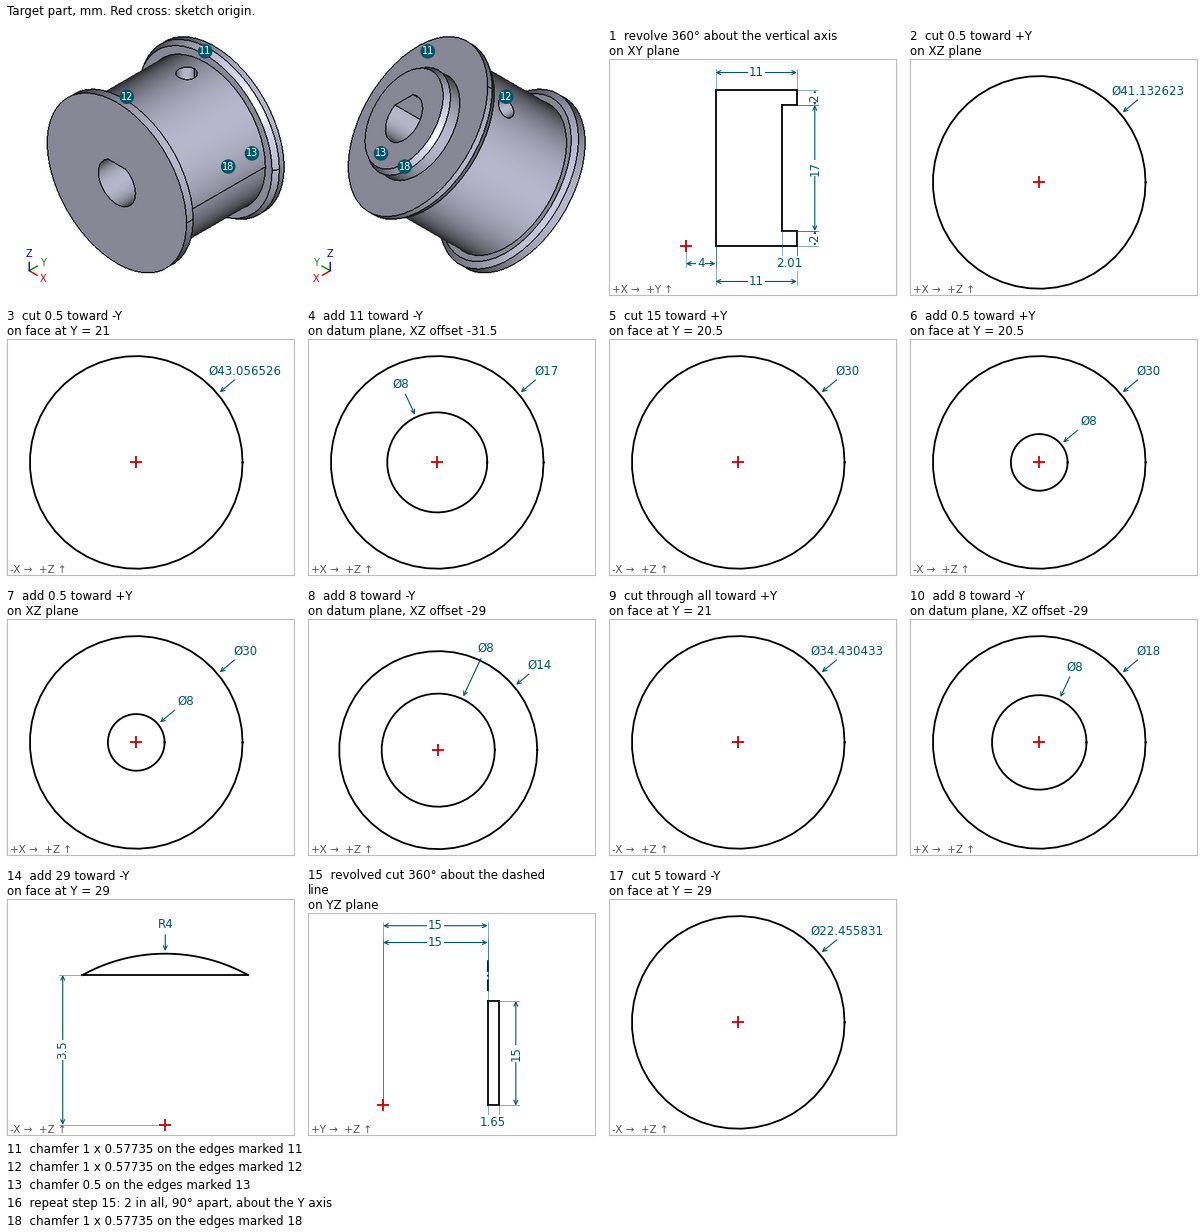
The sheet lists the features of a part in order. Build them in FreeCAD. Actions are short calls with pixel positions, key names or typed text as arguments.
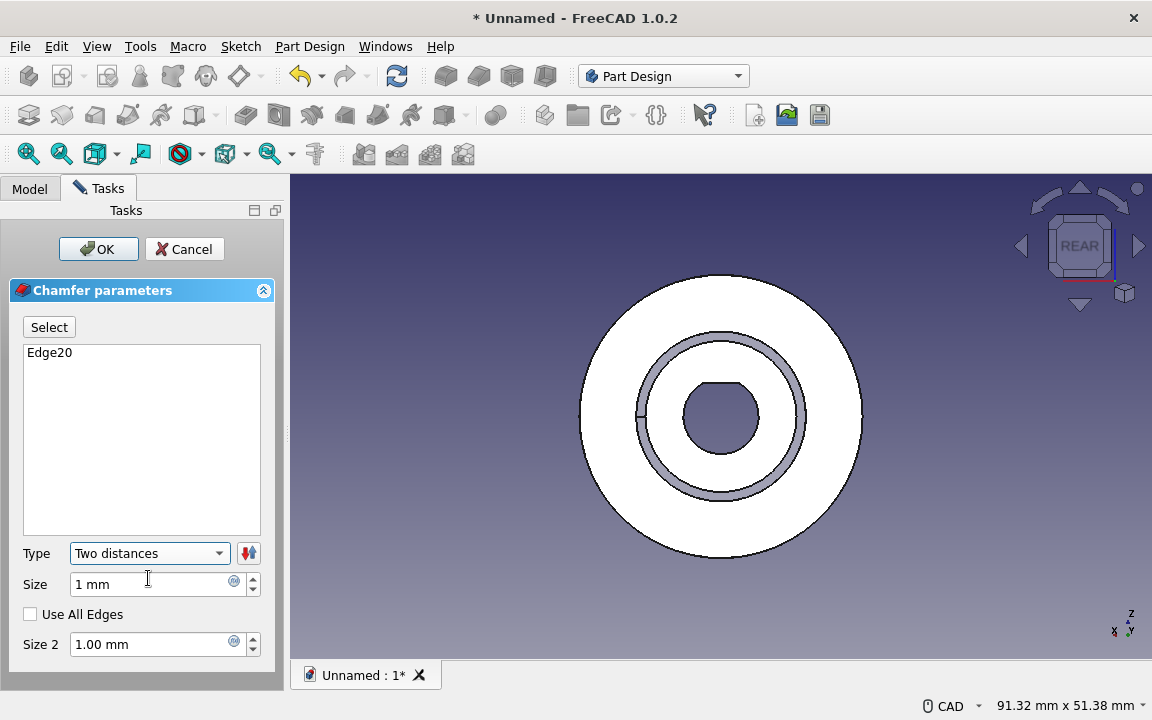
triple_click(158, 644)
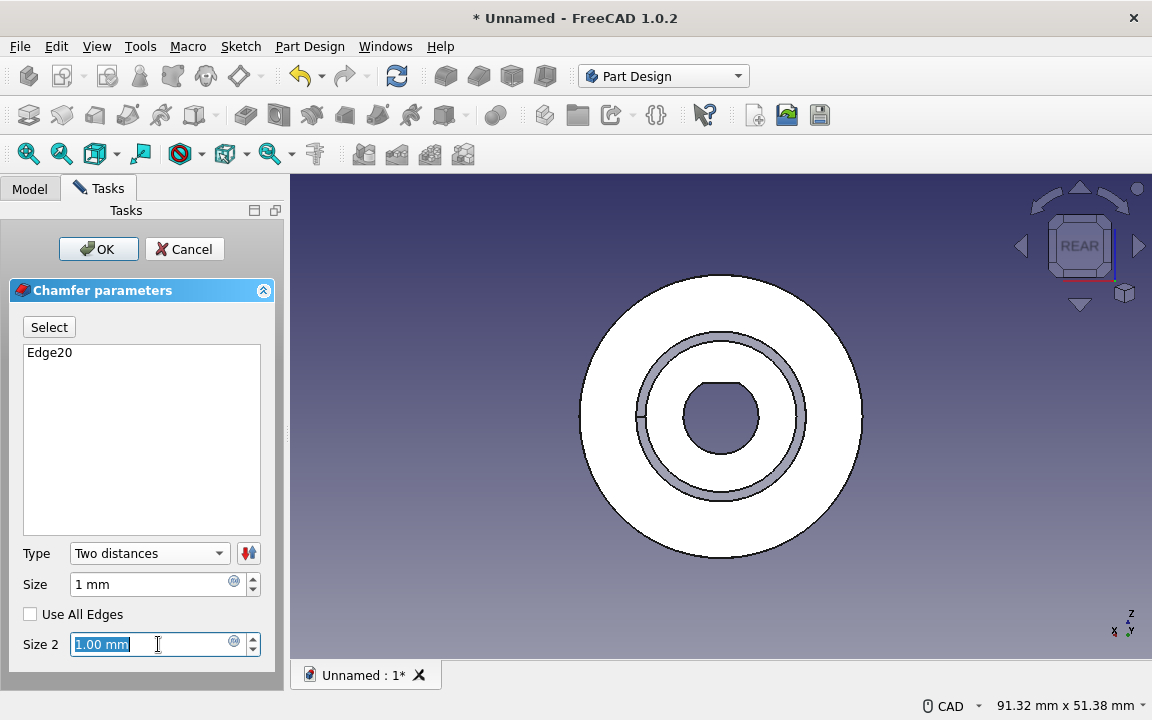
text(0.57735)
key(Tab)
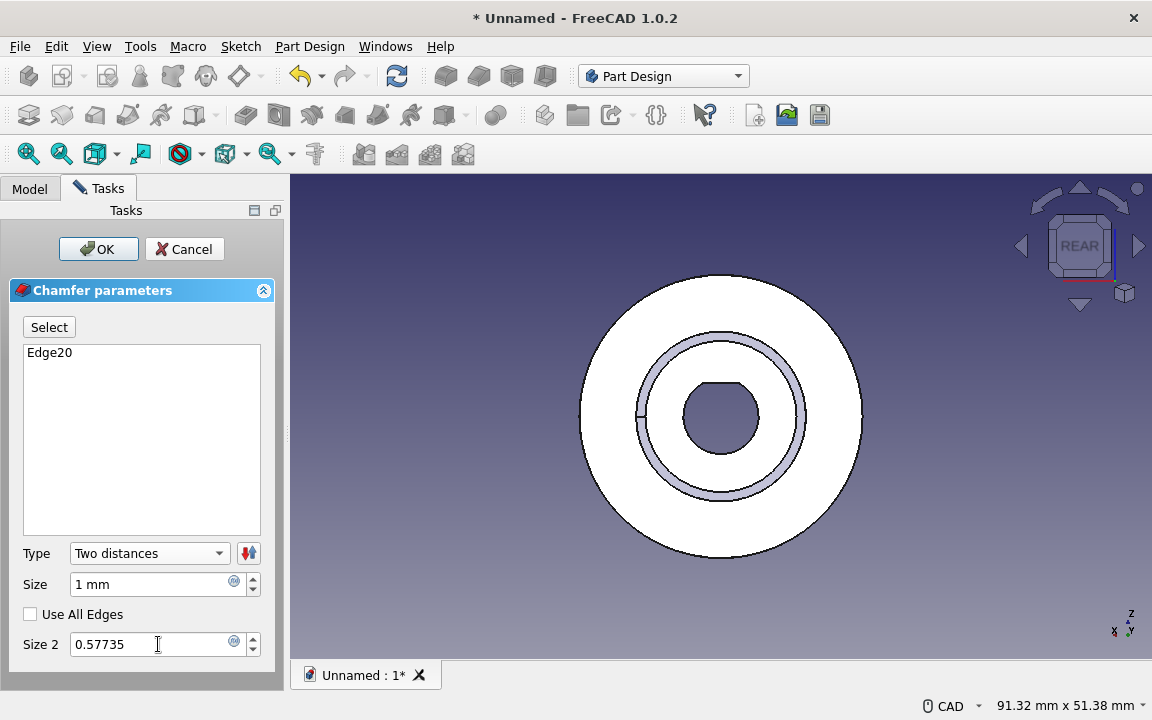
click(249, 554)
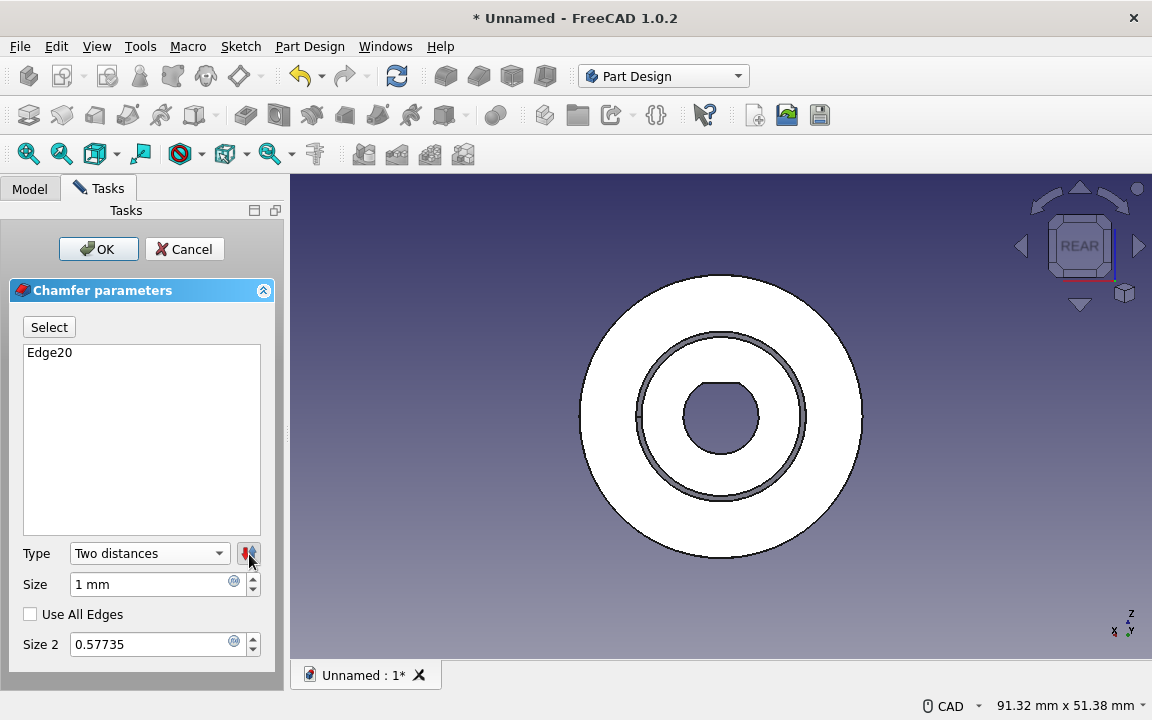
click(99, 249)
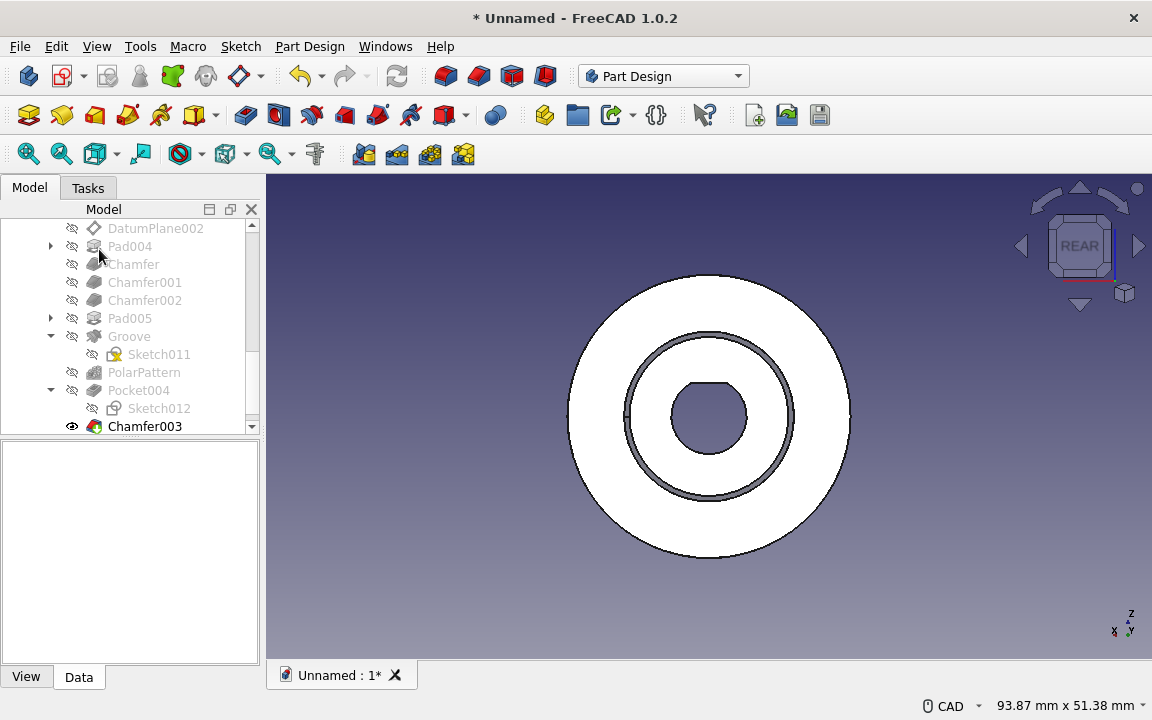
key(0)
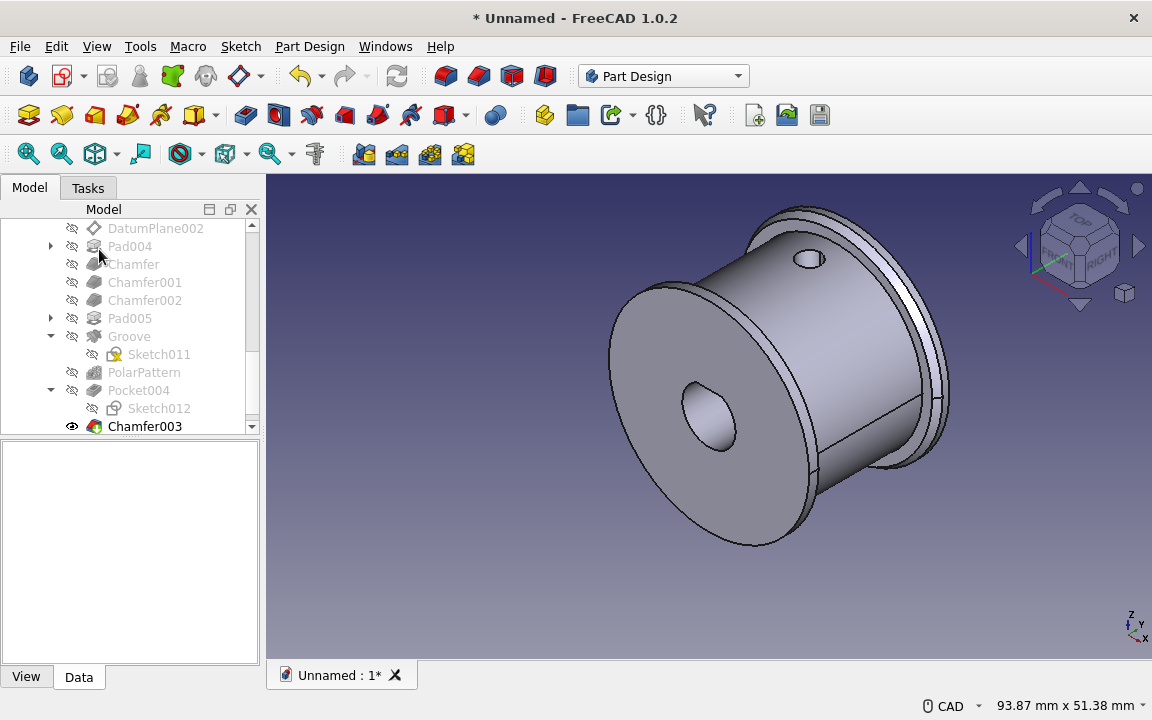
click(29, 154)